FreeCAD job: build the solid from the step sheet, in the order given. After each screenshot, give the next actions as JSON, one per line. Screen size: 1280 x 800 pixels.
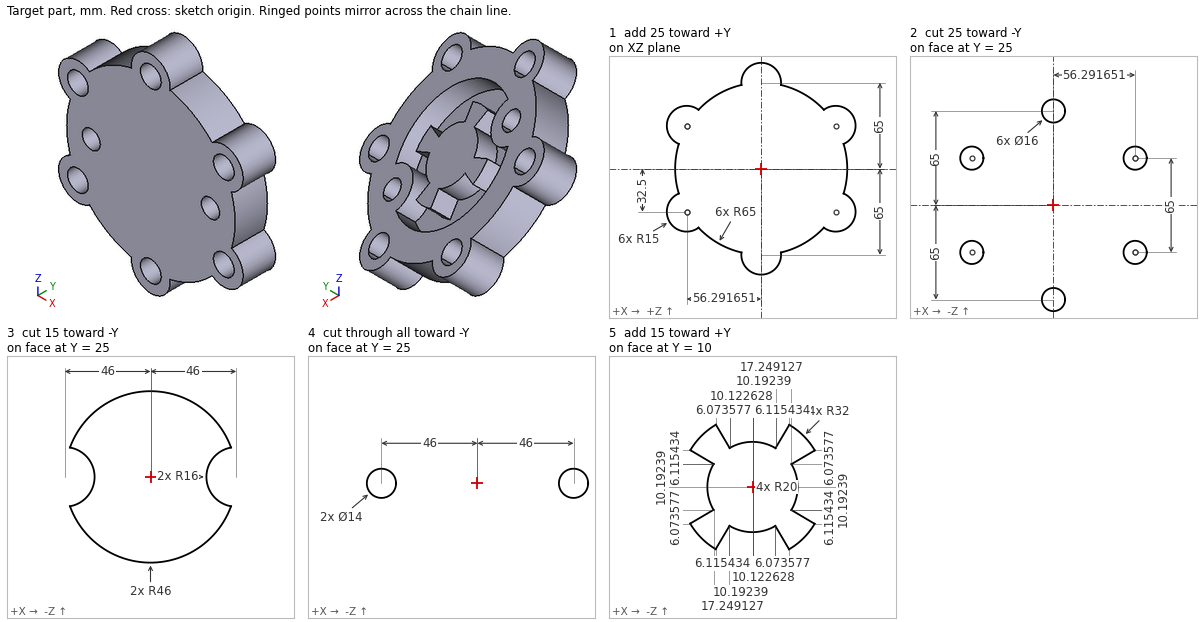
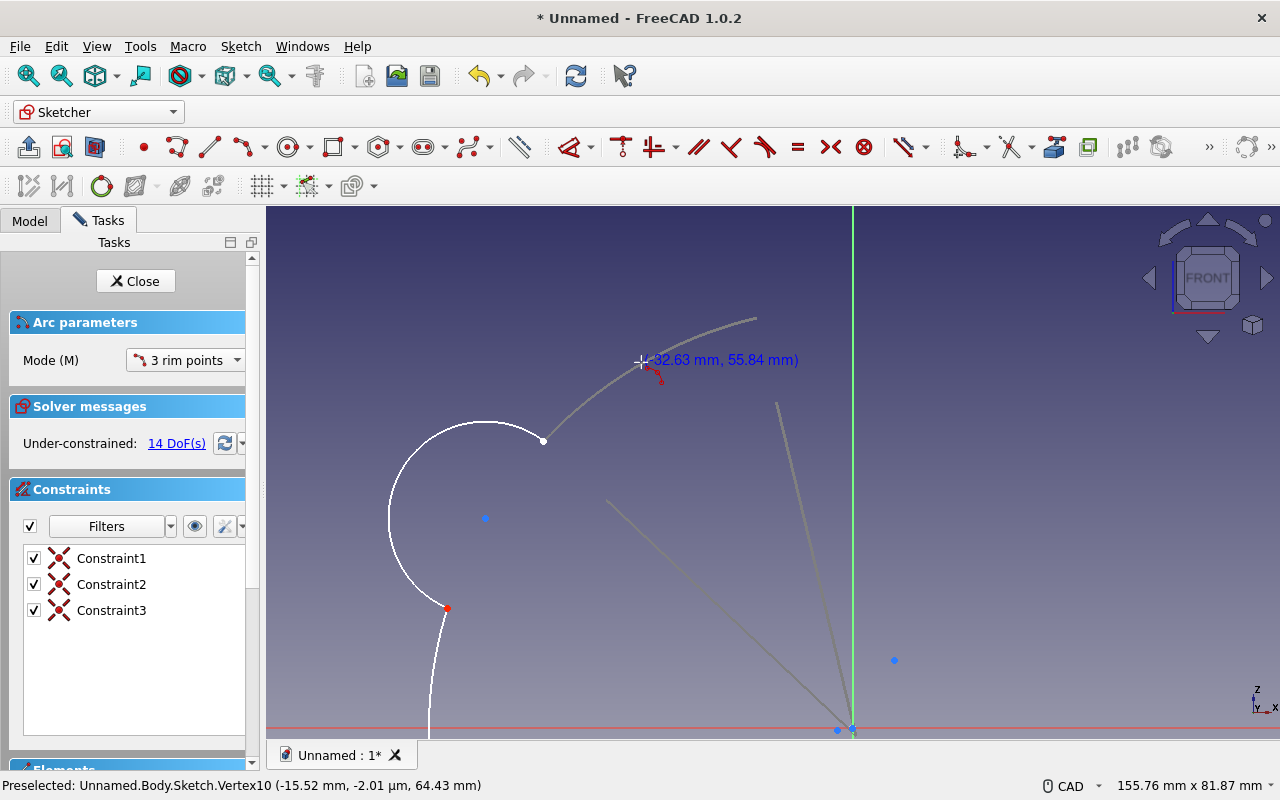
{"action": "left_click", "coordinate": [641, 362]}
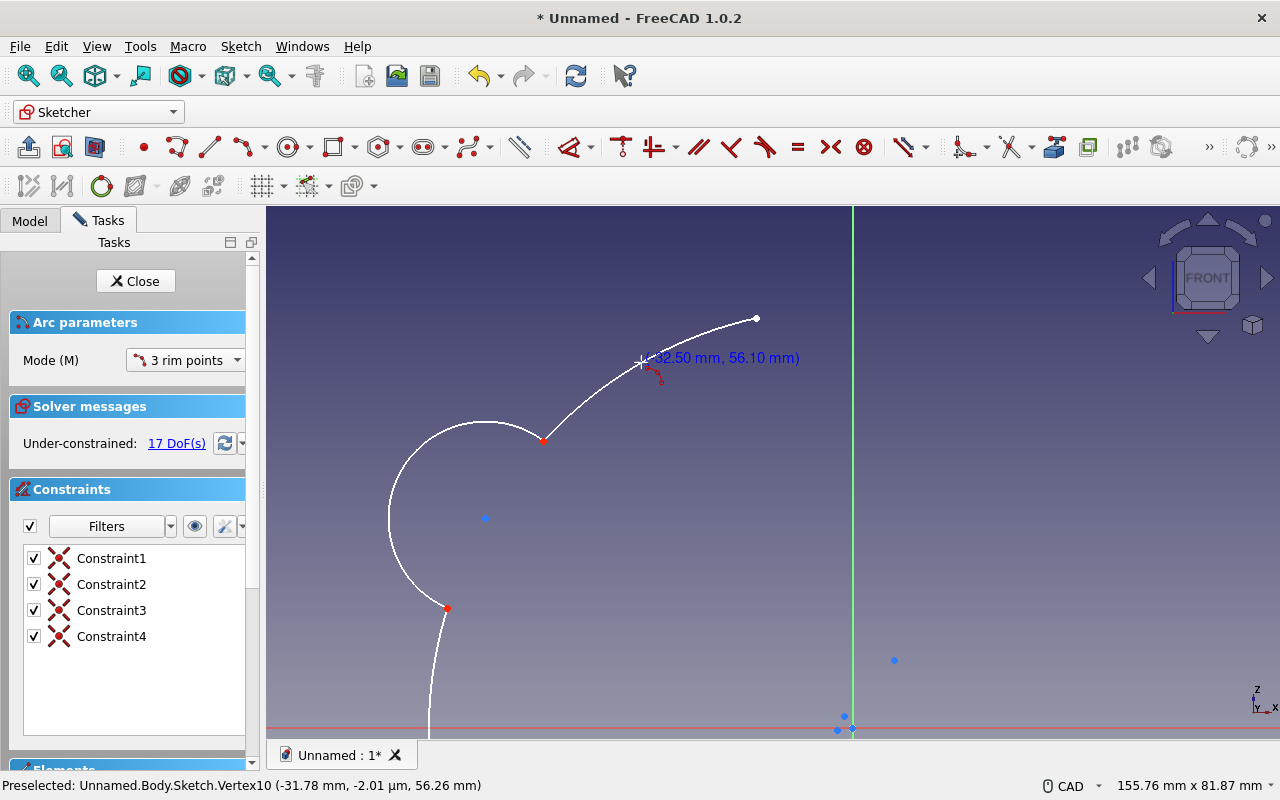
{"action": "left_click", "coordinate": [756, 318]}
{"action": "left_click", "coordinate": [950, 316]}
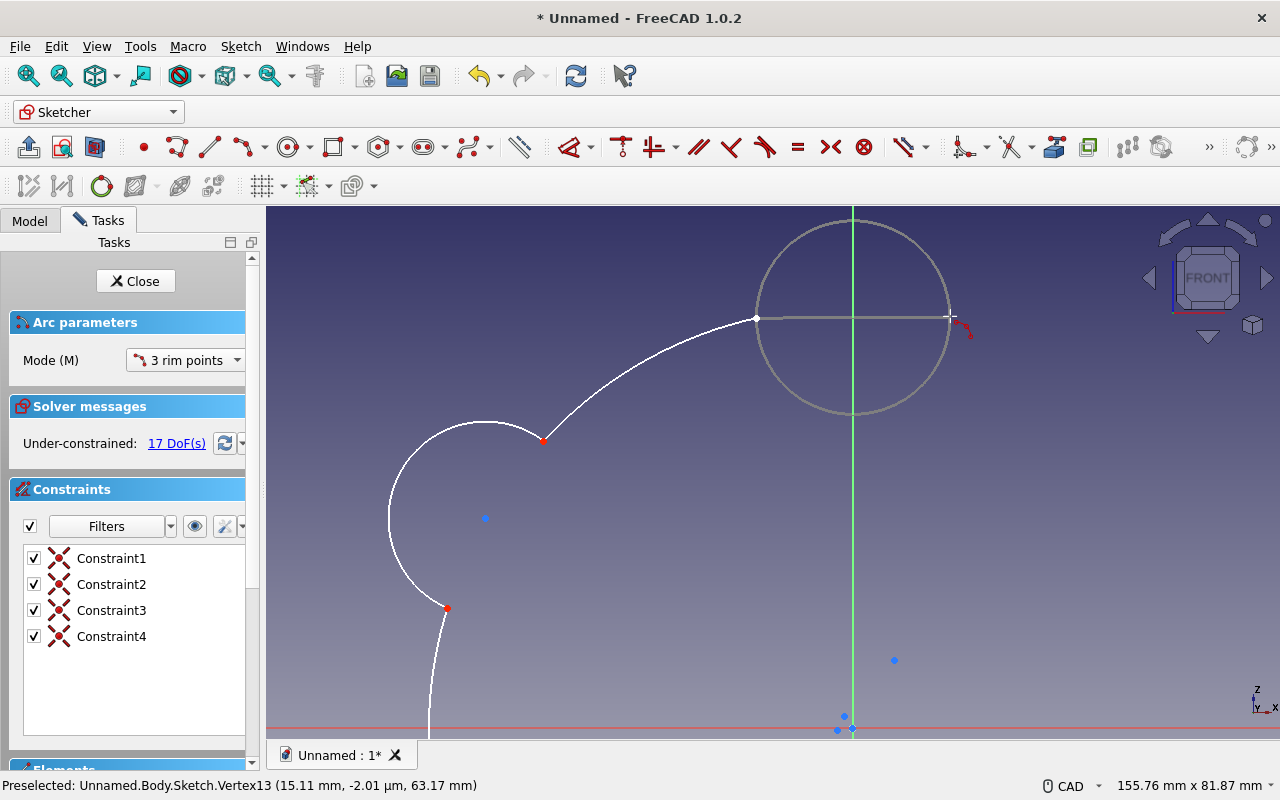
{"action": "scroll", "coordinate": [641, 362], "scroll_direction": "down", "scroll_amount": 6}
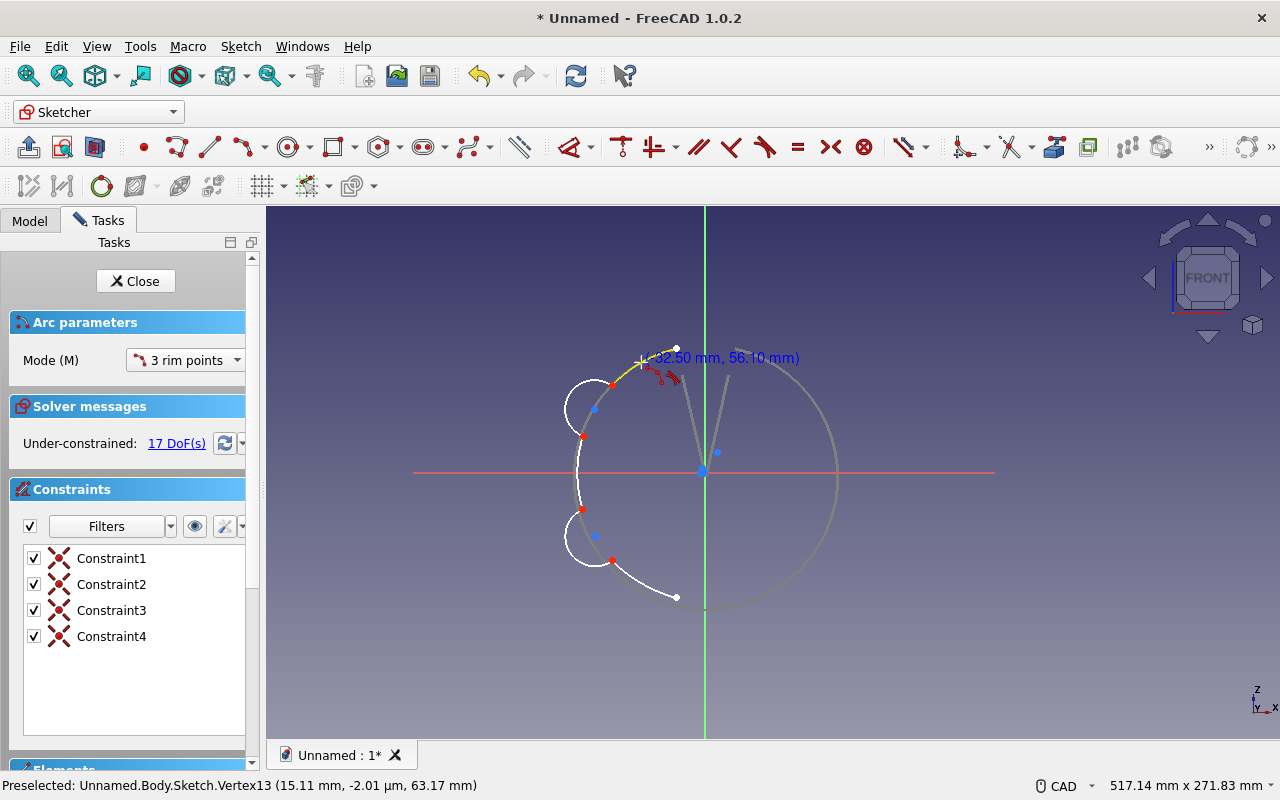
{"action": "left_click", "coordinate": [723, 322]}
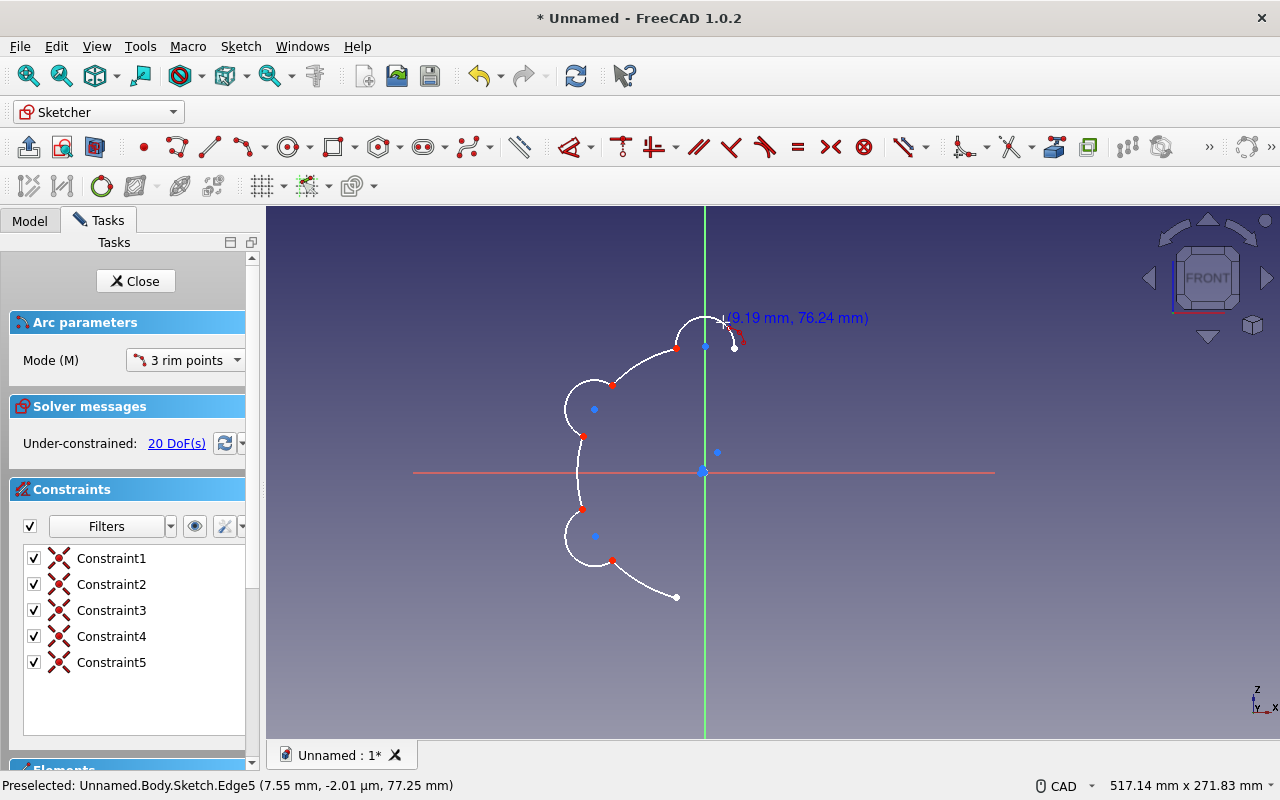
{"action": "left_click", "coordinate": [734, 349]}
{"action": "left_click", "coordinate": [798, 385]}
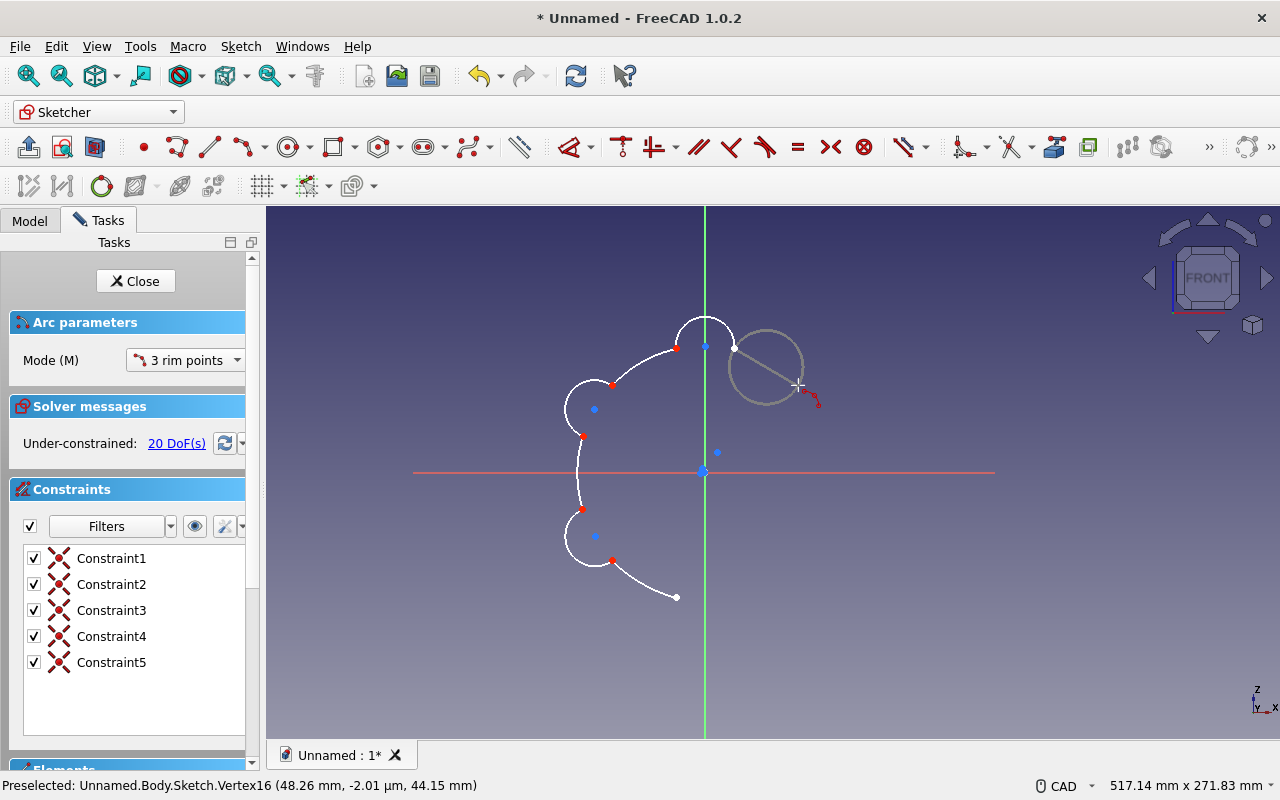
{"action": "scroll", "coordinate": [769, 362], "scroll_direction": "up", "scroll_amount": 6}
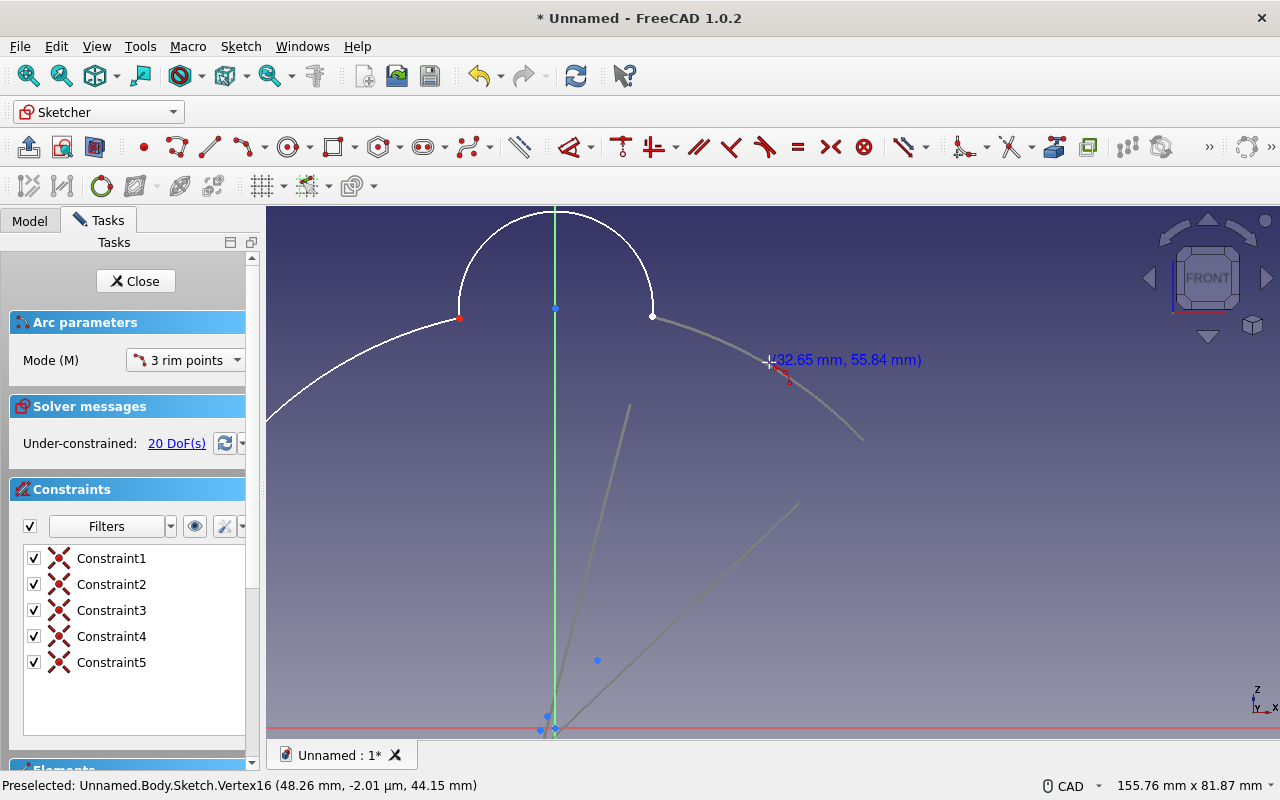
{"action": "left_click", "coordinate": [767, 362]}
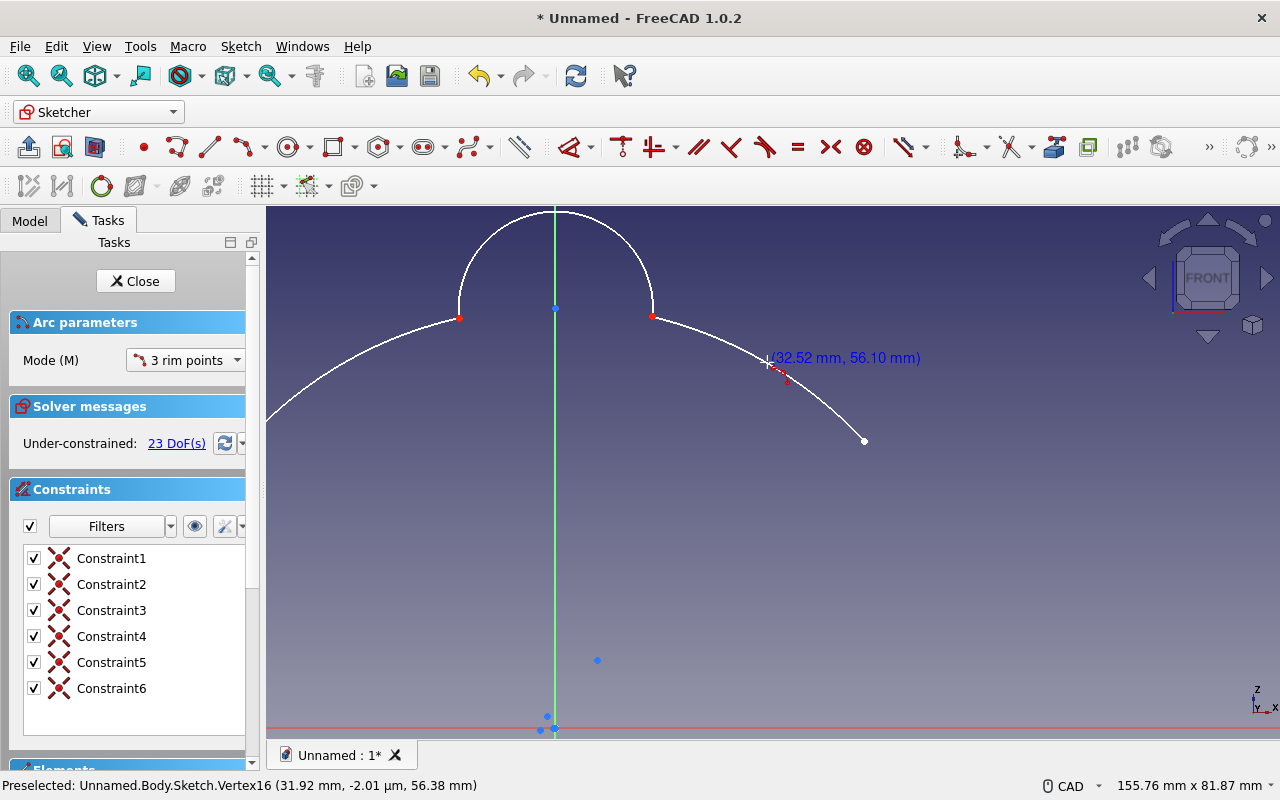
{"action": "left_click", "coordinate": [864, 441]}
{"action": "left_click", "coordinate": [960, 606]}
{"action": "left_click", "coordinate": [1006, 468]}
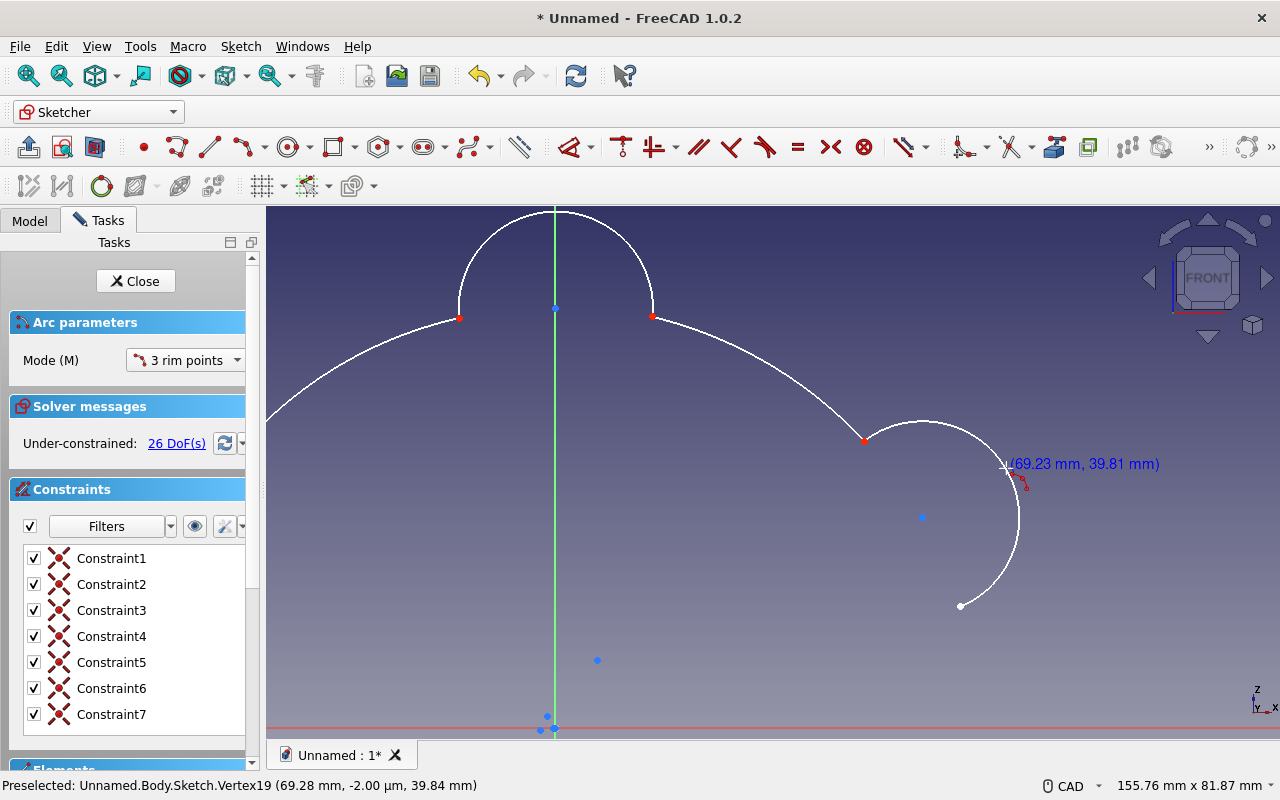
{"action": "left_click", "coordinate": [960, 607]}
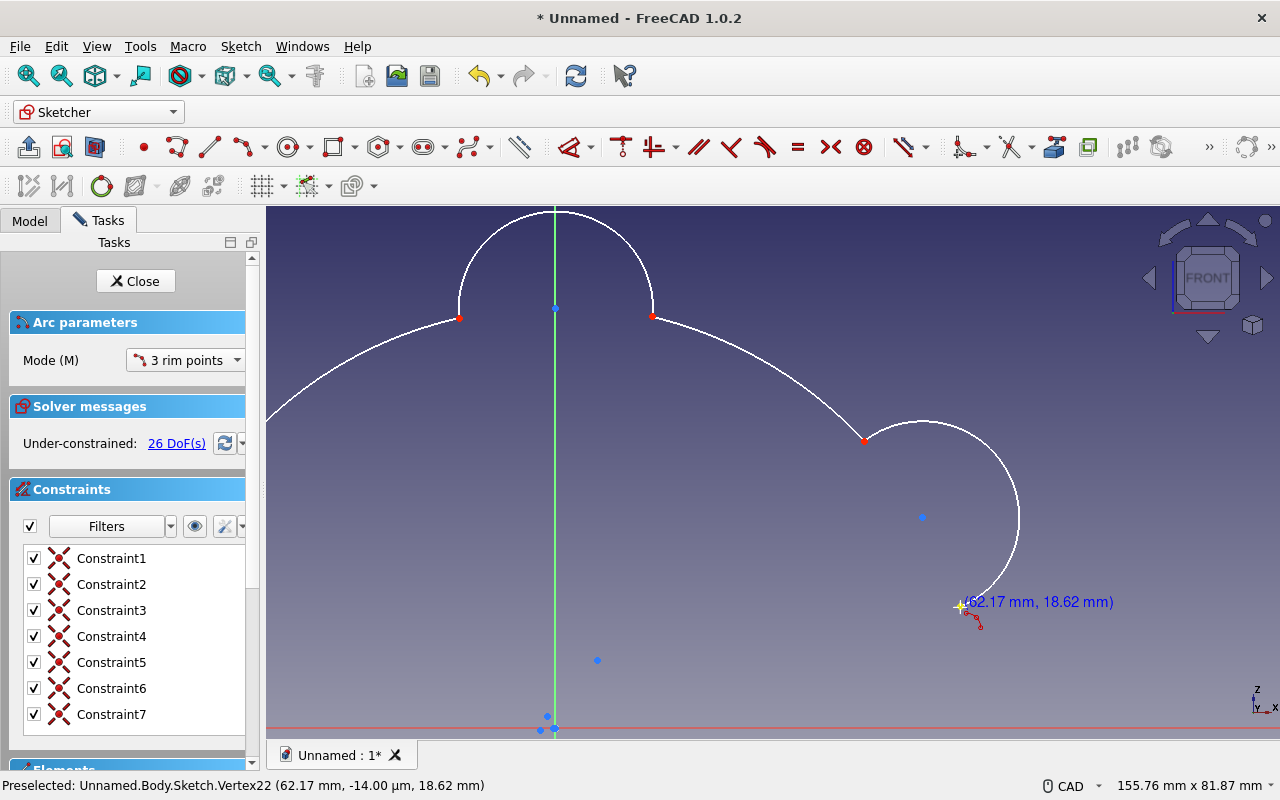
{"action": "scroll", "coordinate": [769, 362], "scroll_direction": "down", "scroll_amount": 6}